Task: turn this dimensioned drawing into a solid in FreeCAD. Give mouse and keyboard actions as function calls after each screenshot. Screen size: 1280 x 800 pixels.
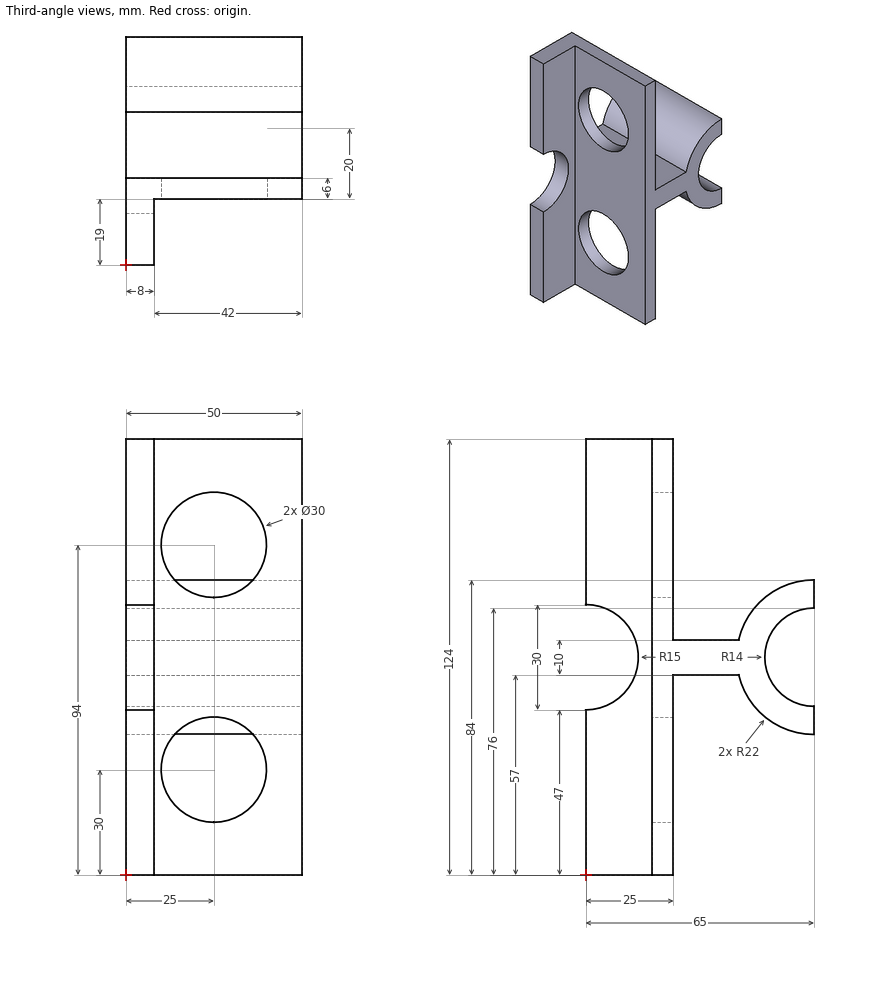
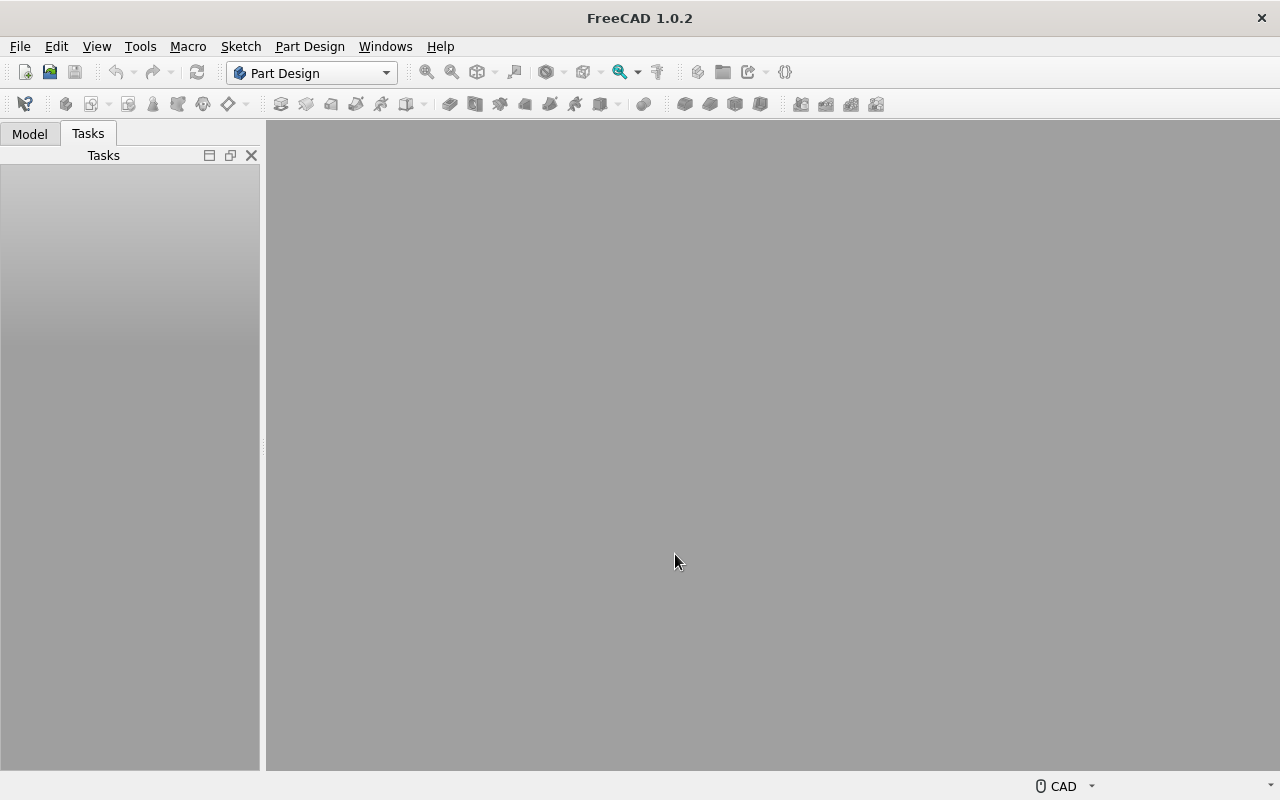
key(ctrl+n)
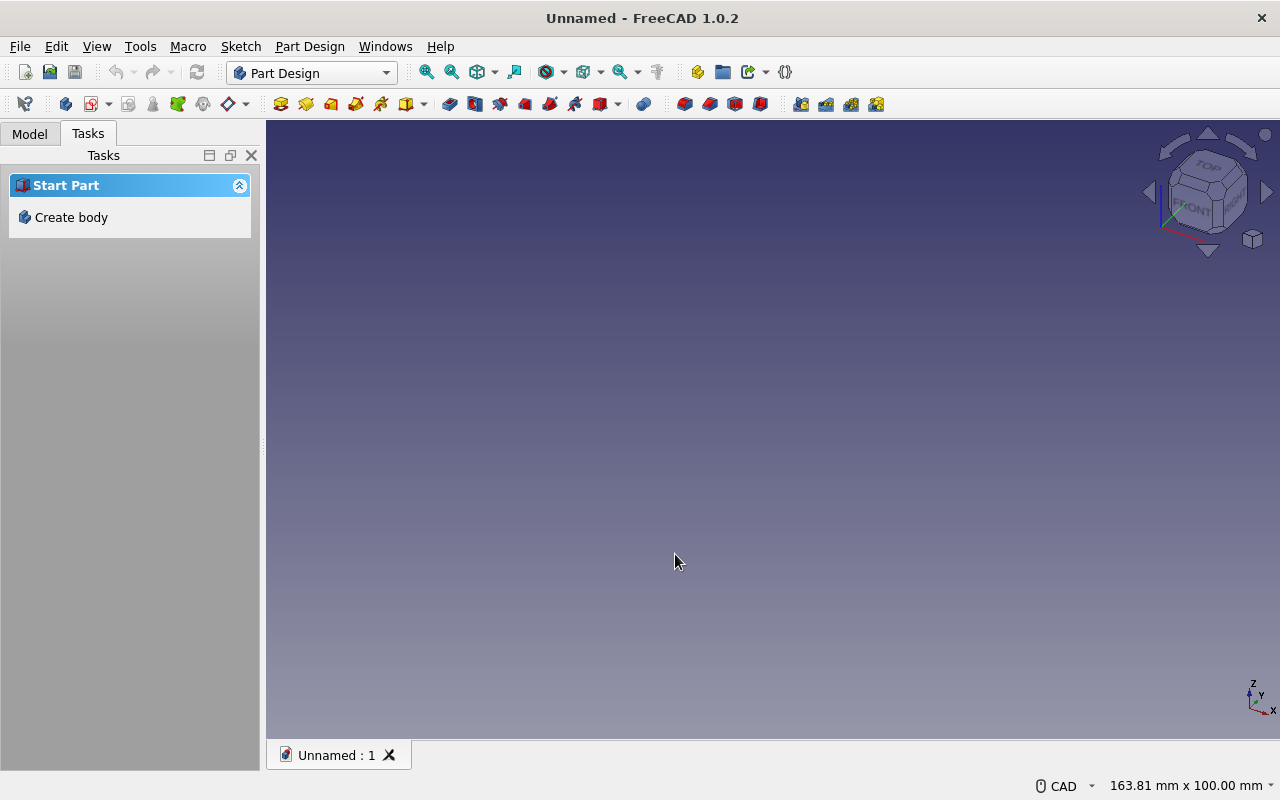
click(90, 104)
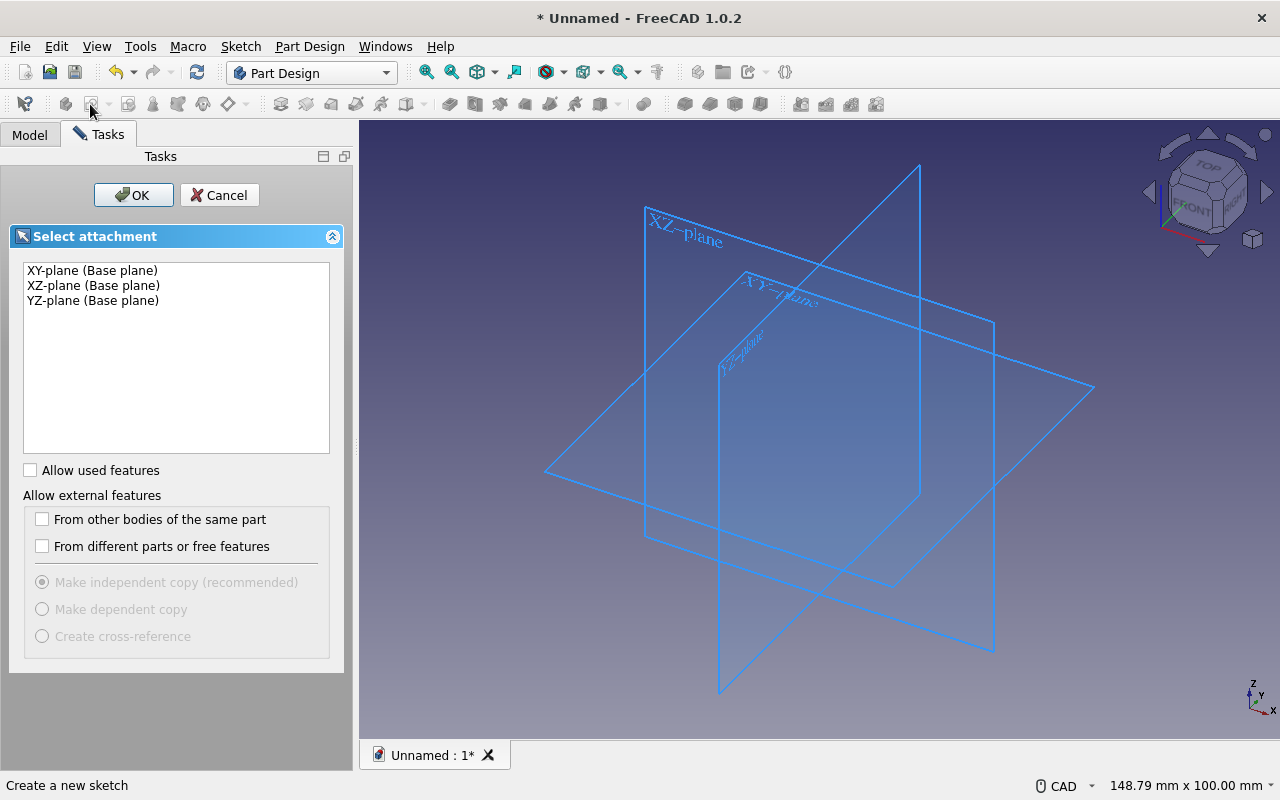
click(84, 270)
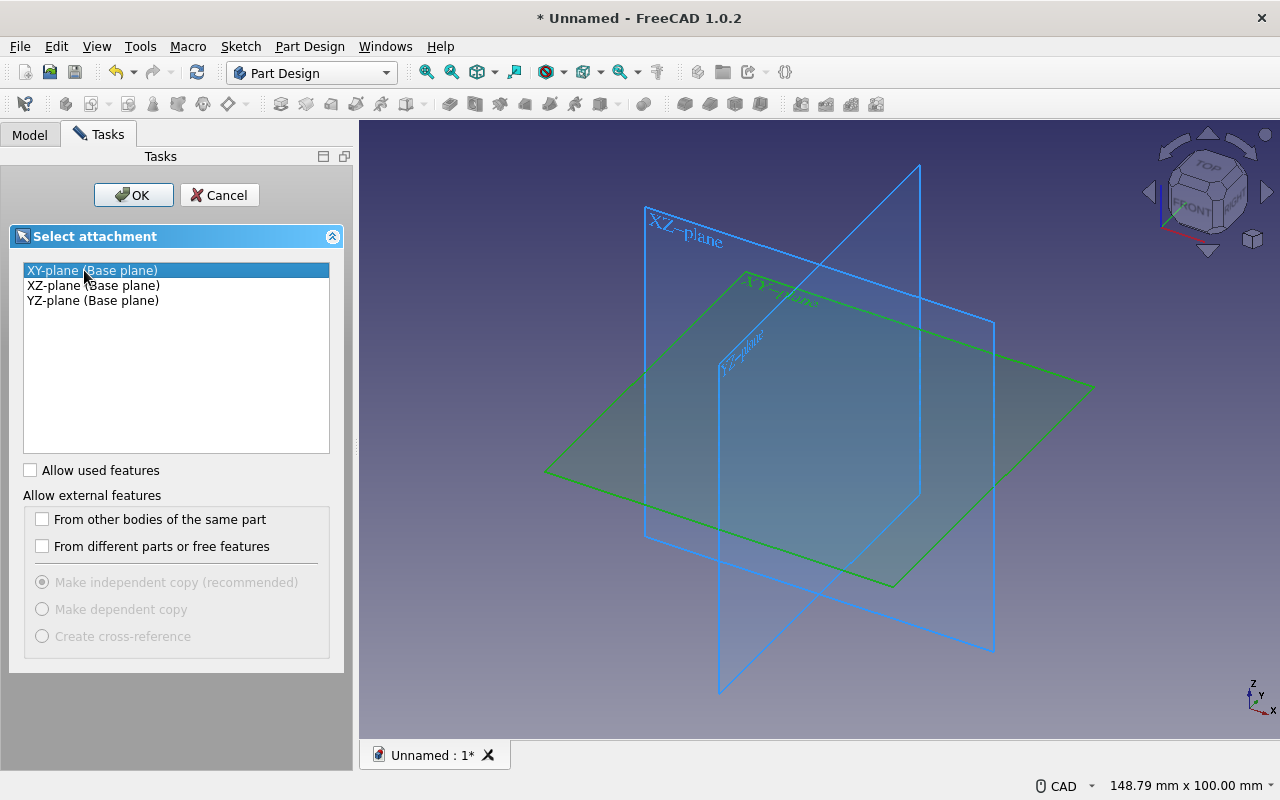
click(134, 195)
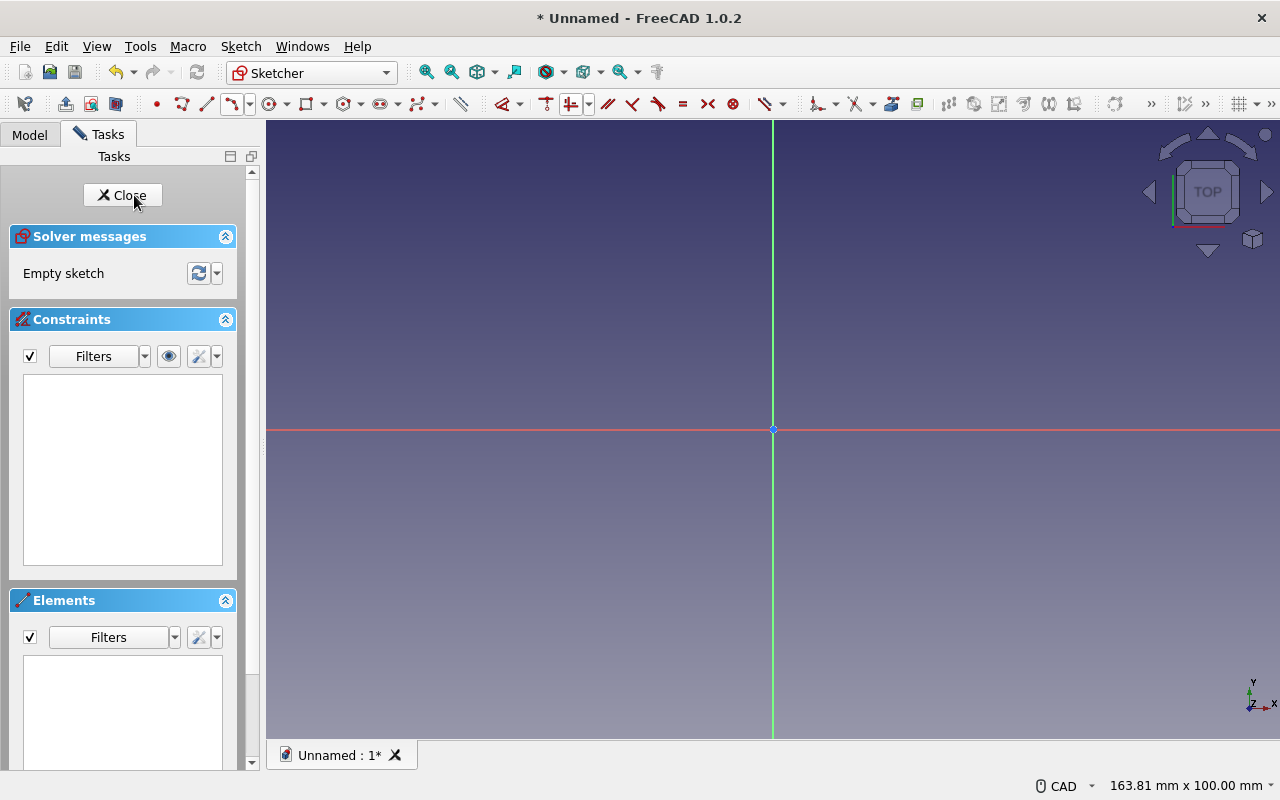
scroll(1115, 258, up, 3)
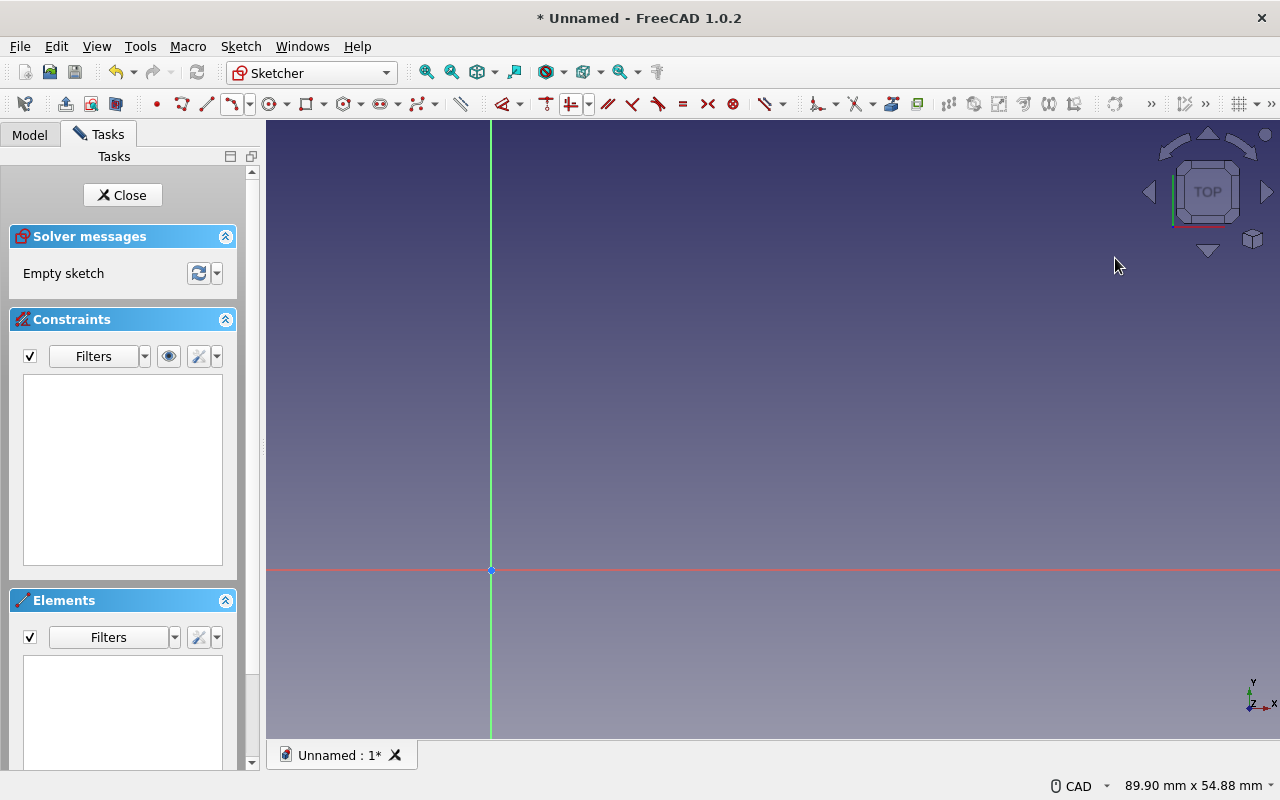
key(g)
key(m)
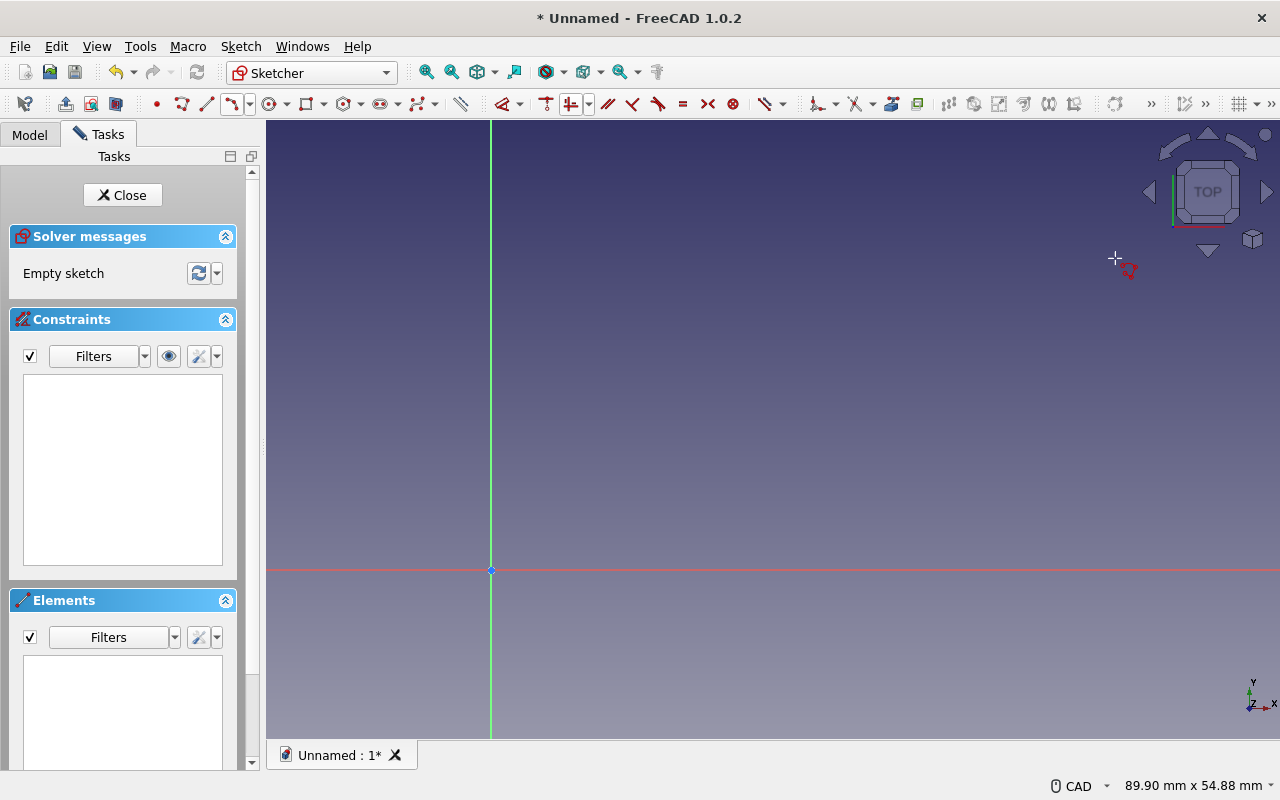
click(491, 570)
click(581, 561)
click(581, 356)
click(1055, 356)
click(1055, 288)
click(500, 288)
click(491, 570)
key(Escape)
key(Escape)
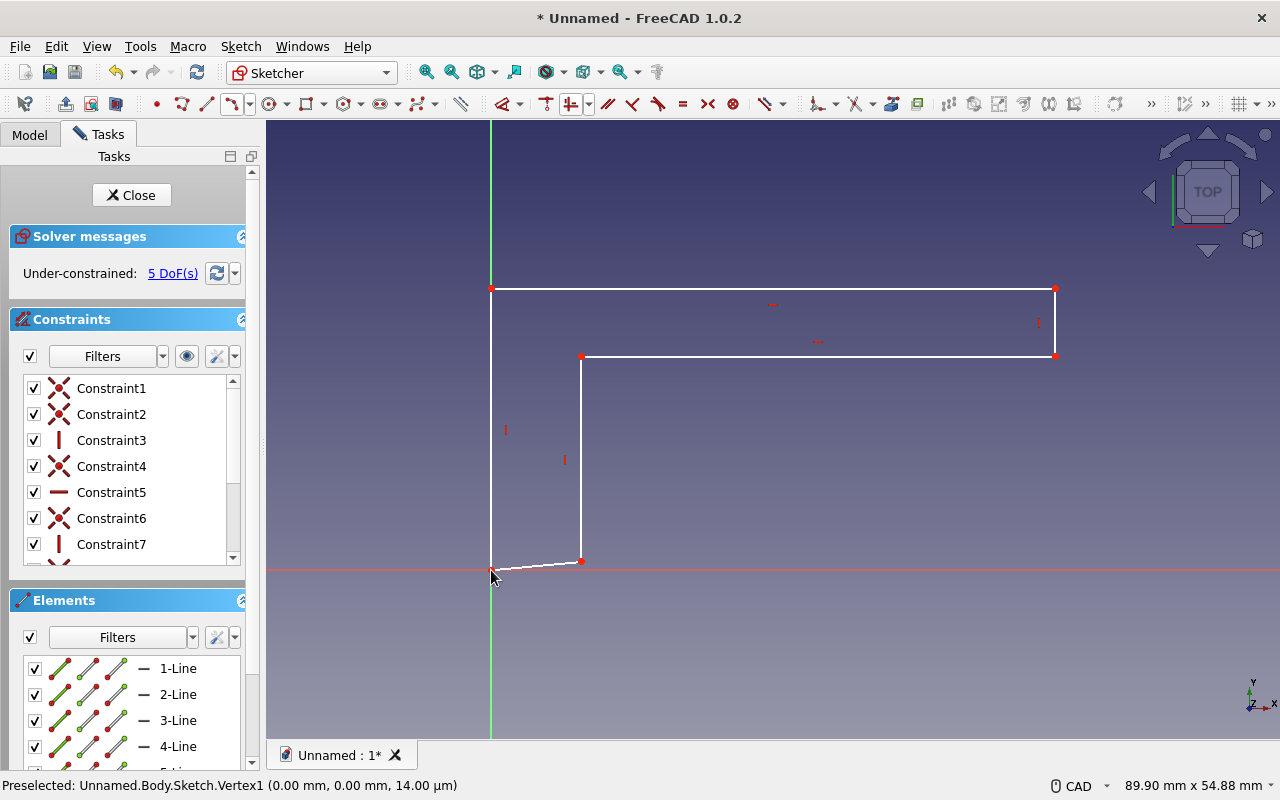
click(518, 568)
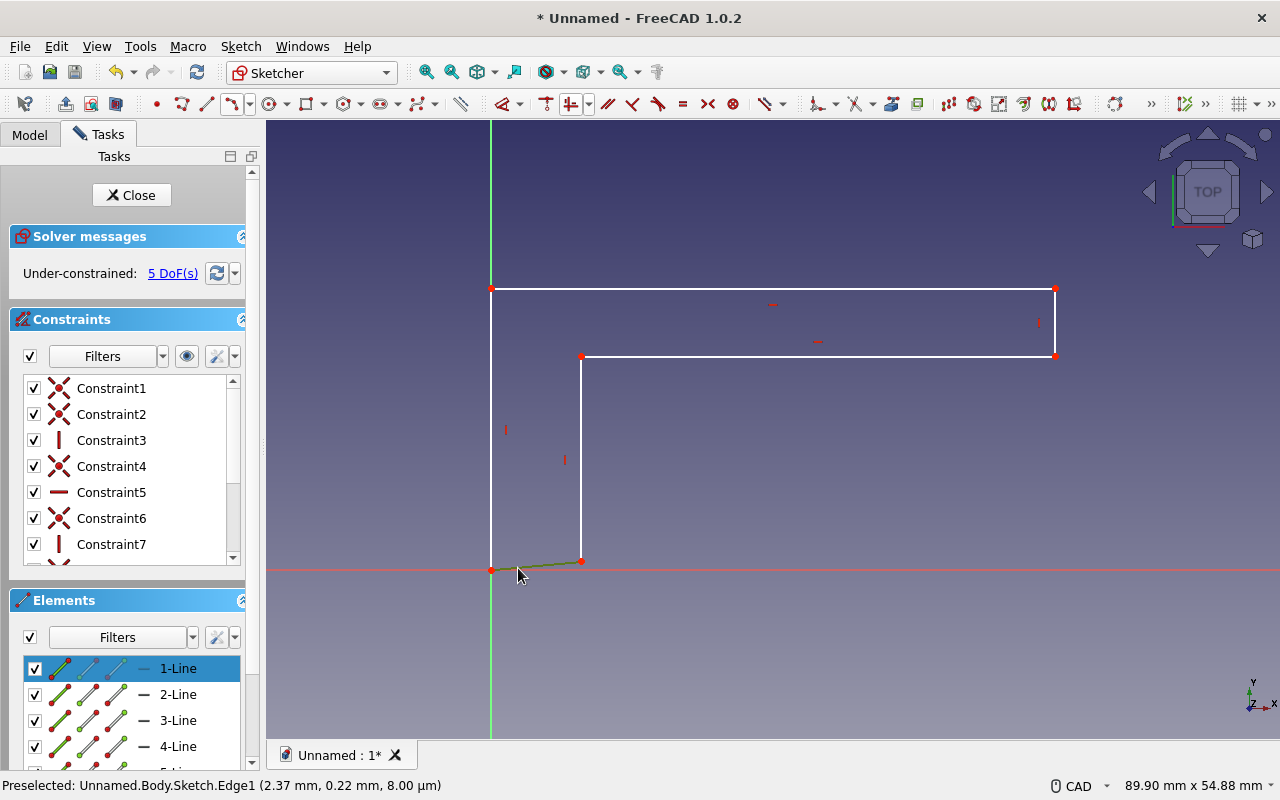
key(h)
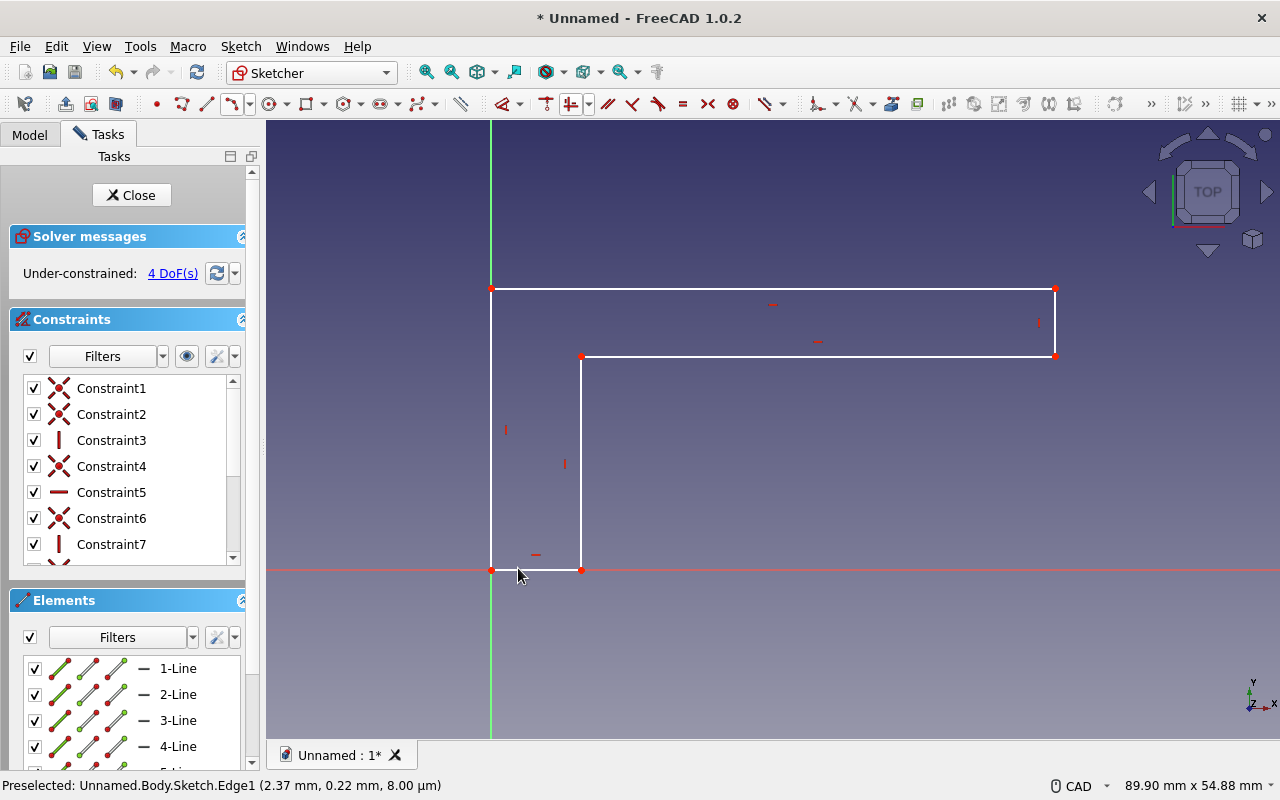
key(d)